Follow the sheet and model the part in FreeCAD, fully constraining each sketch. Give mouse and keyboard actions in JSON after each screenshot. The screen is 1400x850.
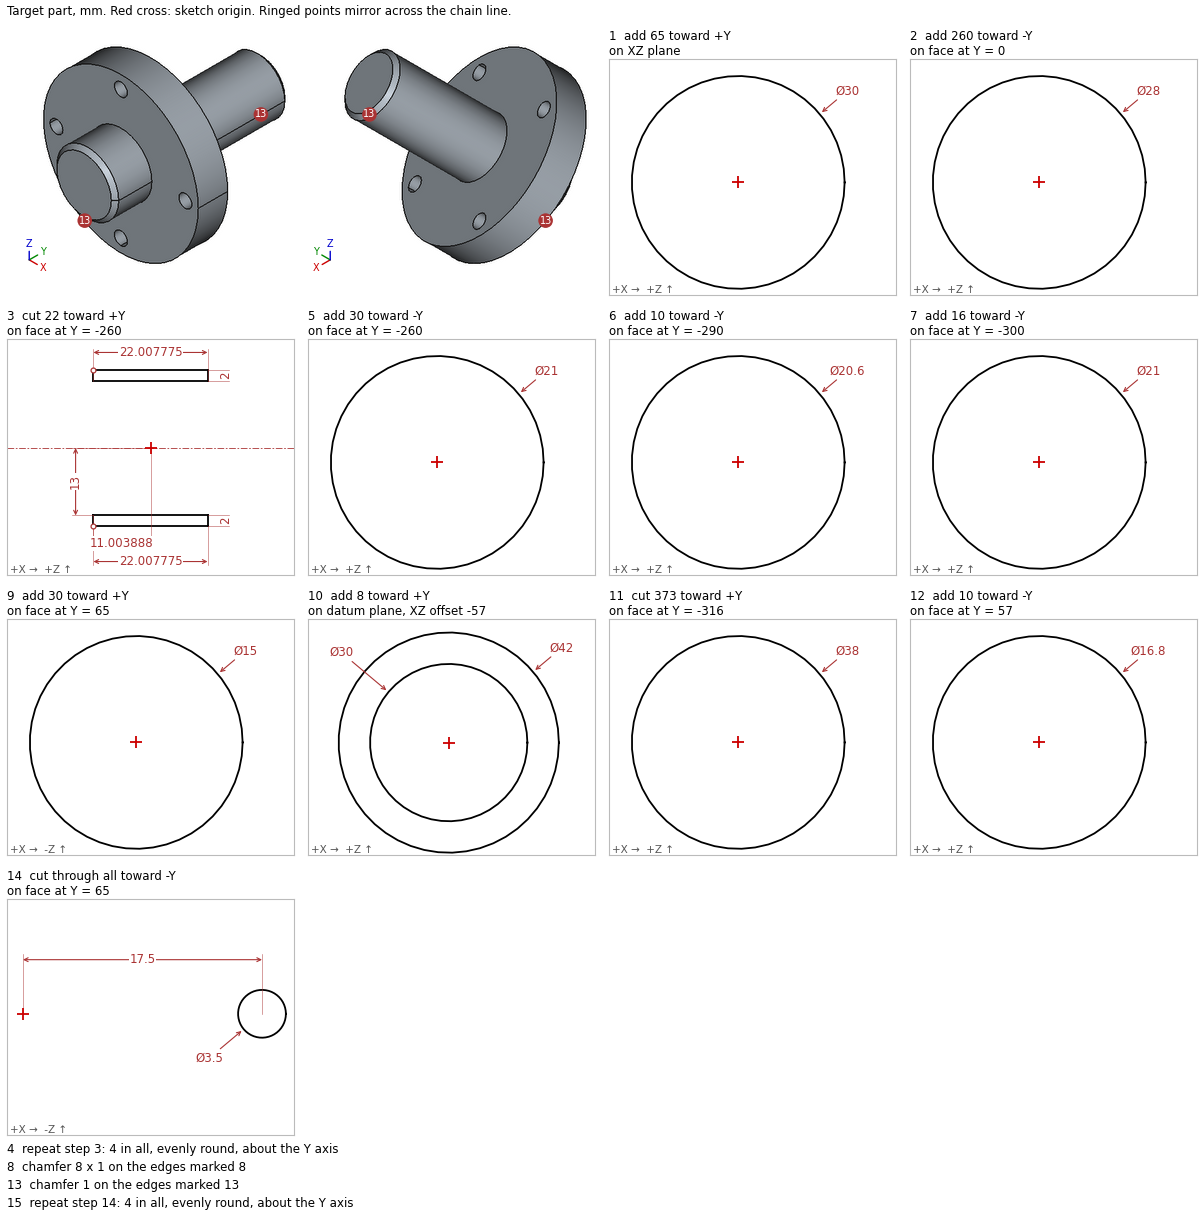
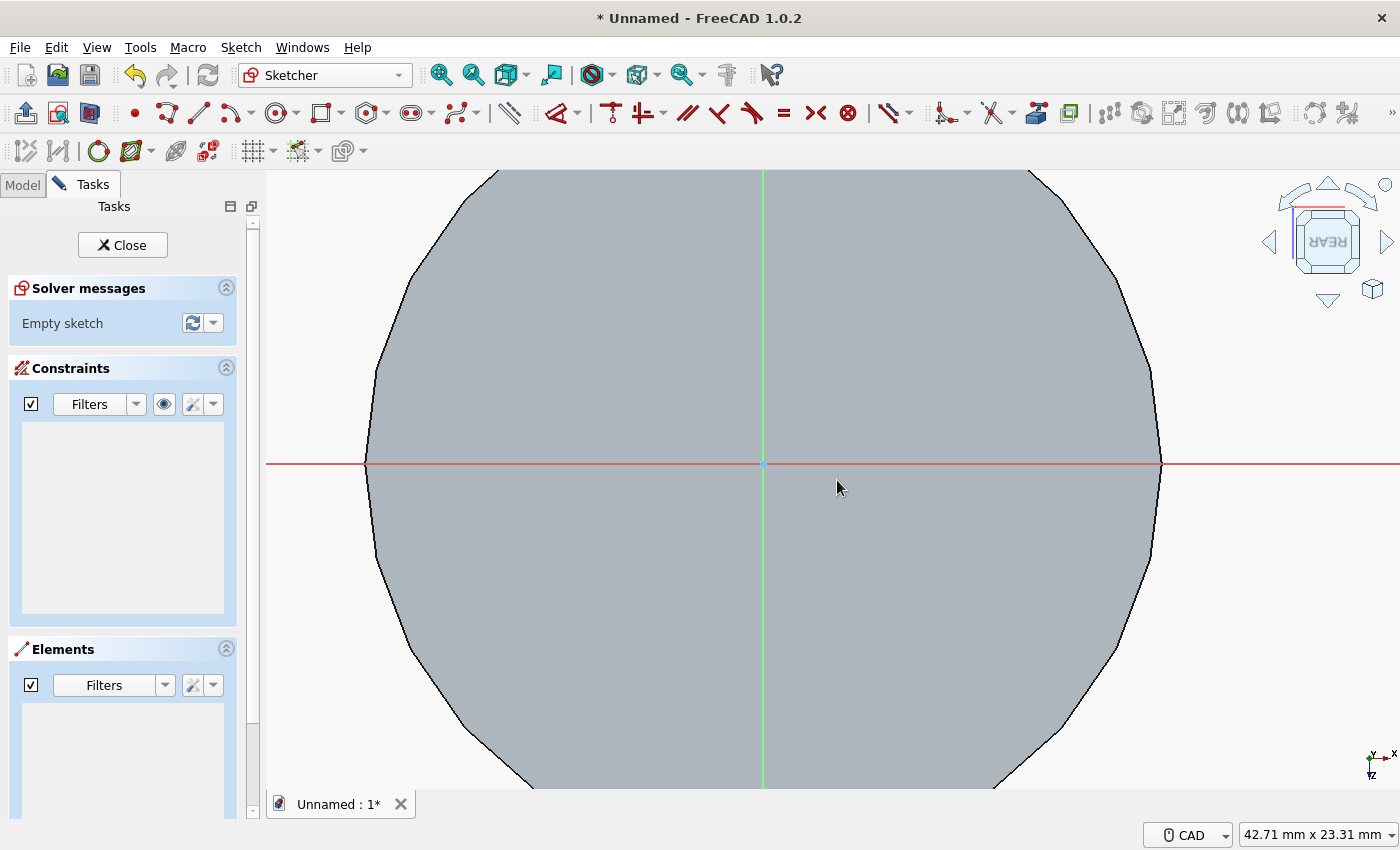
{"action": "key", "text": "g c"}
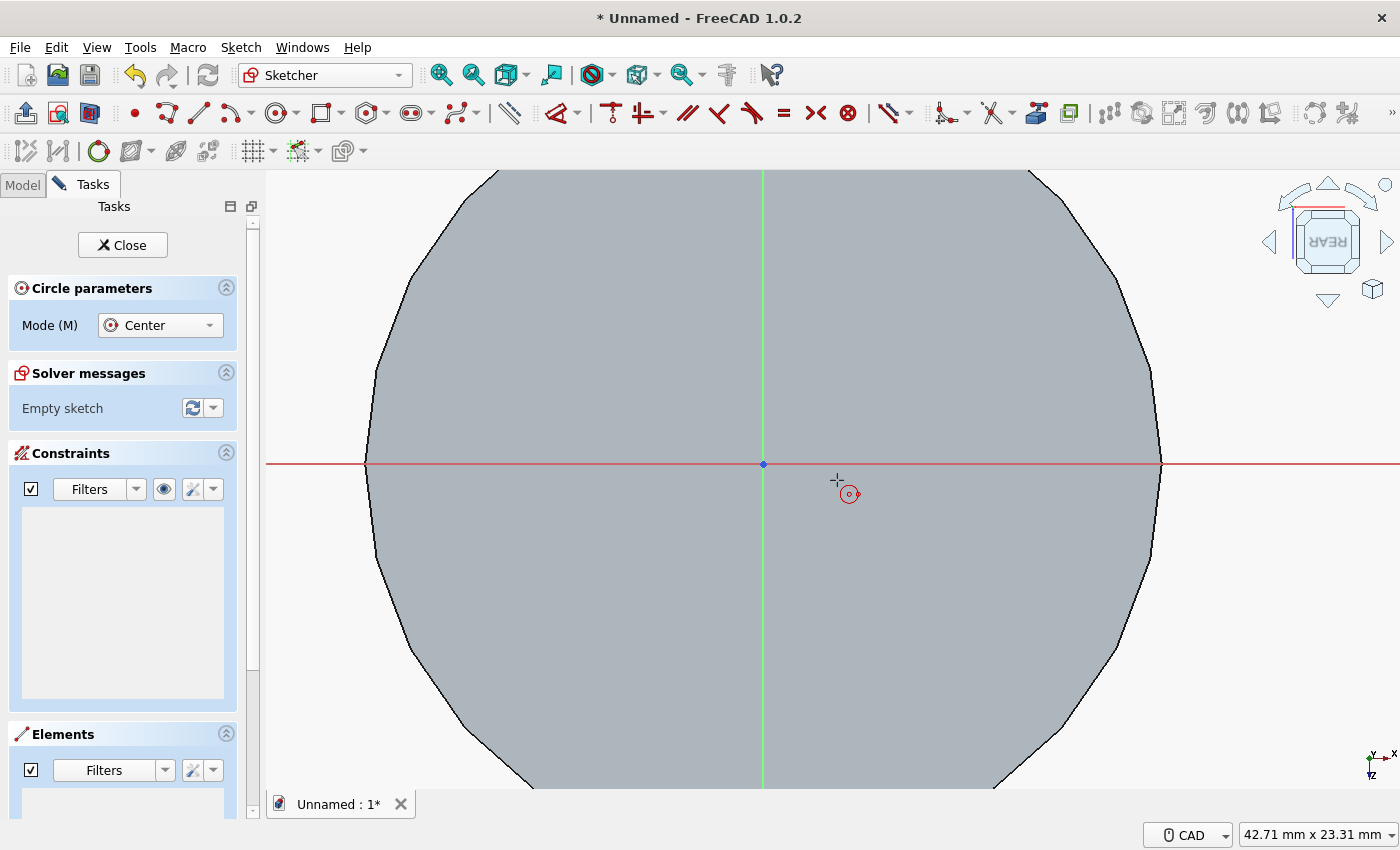
{"action": "left_click", "coordinate": [763, 464]}
{"action": "mouse_move", "coordinate": [904, 323]}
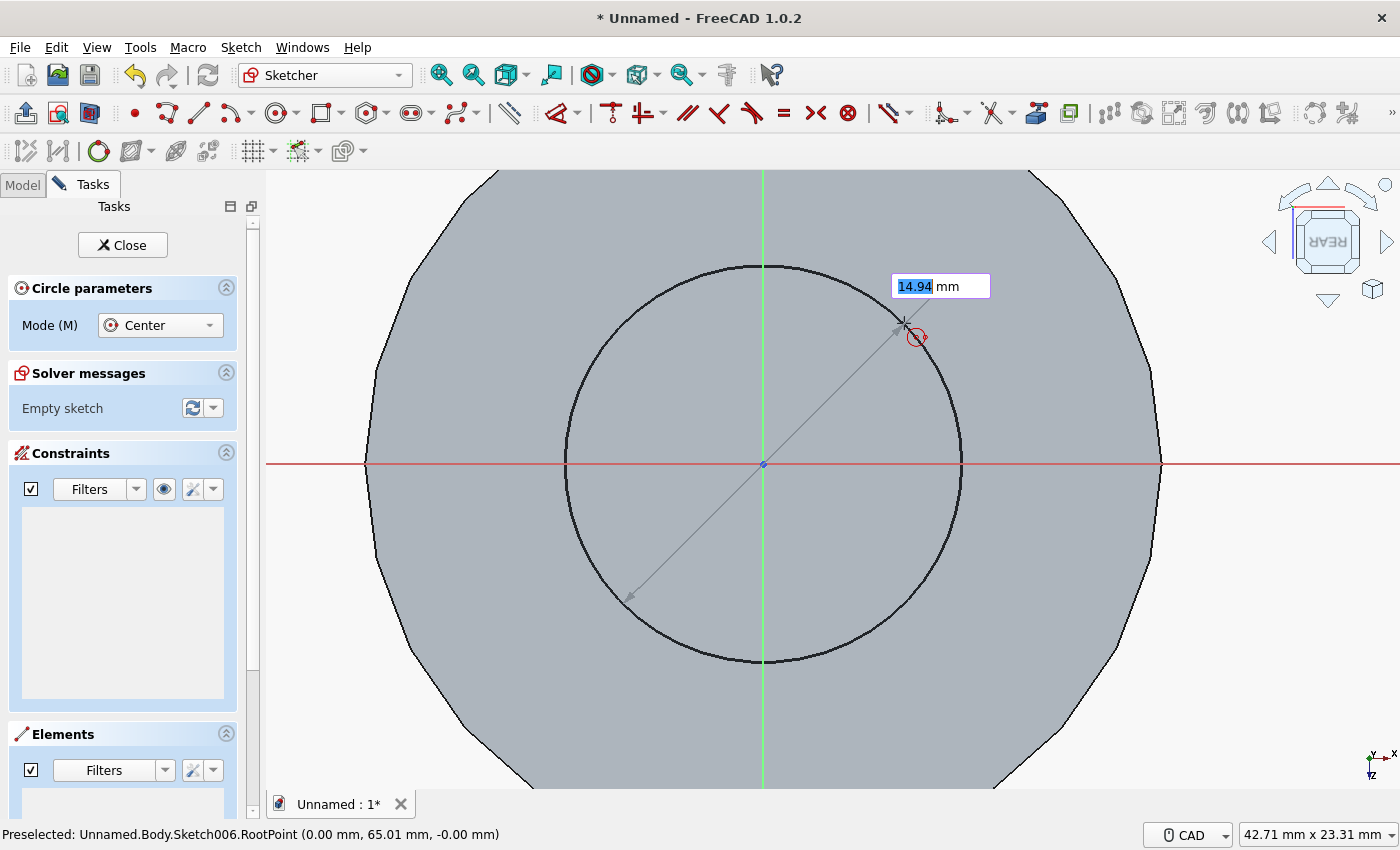
{"action": "type", "text": "15"}
{"action": "key", "text": "Return"}
{"action": "key", "text": "Escape"}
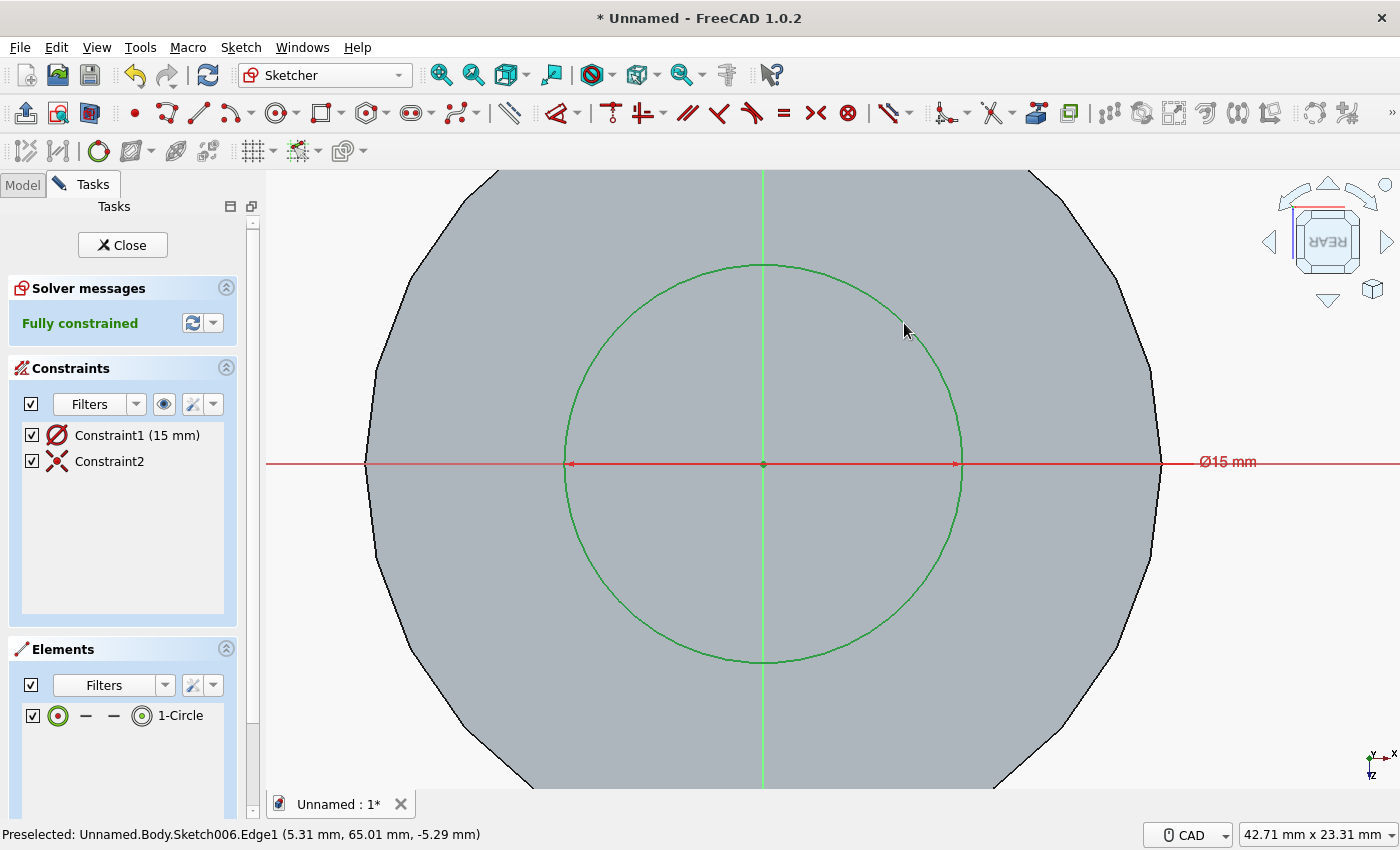
{"action": "left_click", "coordinate": [123, 245]}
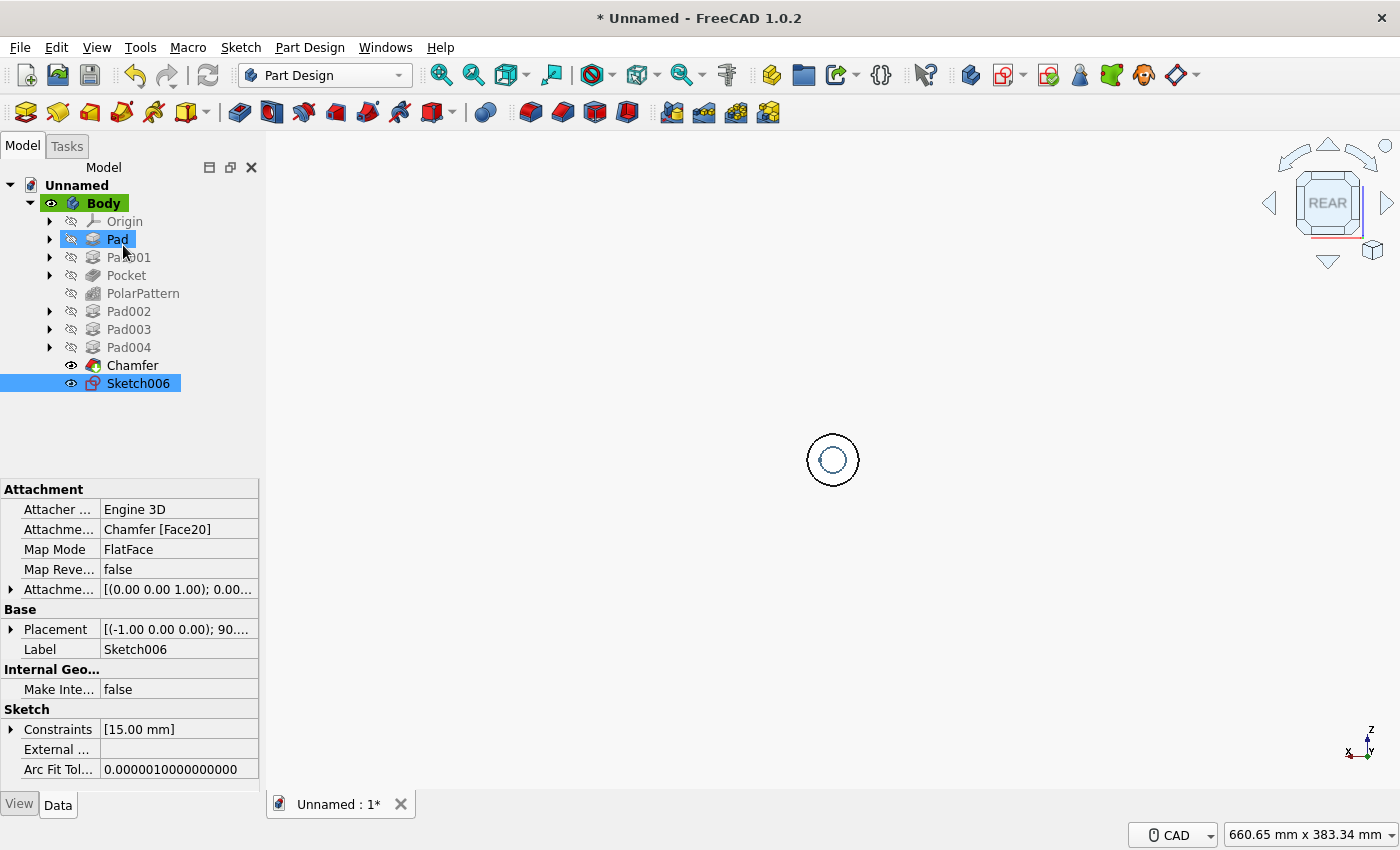
{"action": "left_click", "coordinate": [26, 112]}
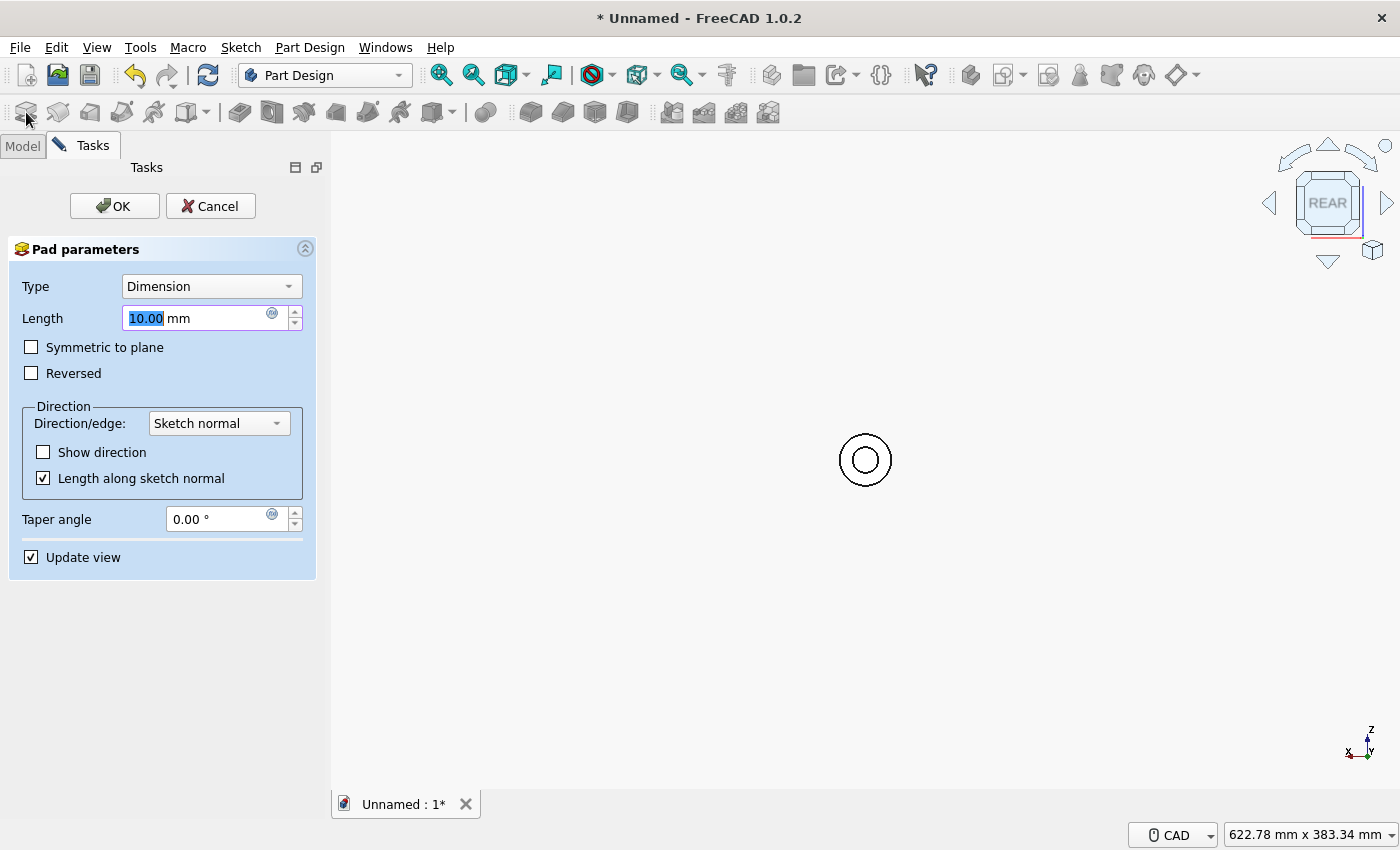
{"action": "type", "text": "30"}
{"action": "key", "text": "Tab"}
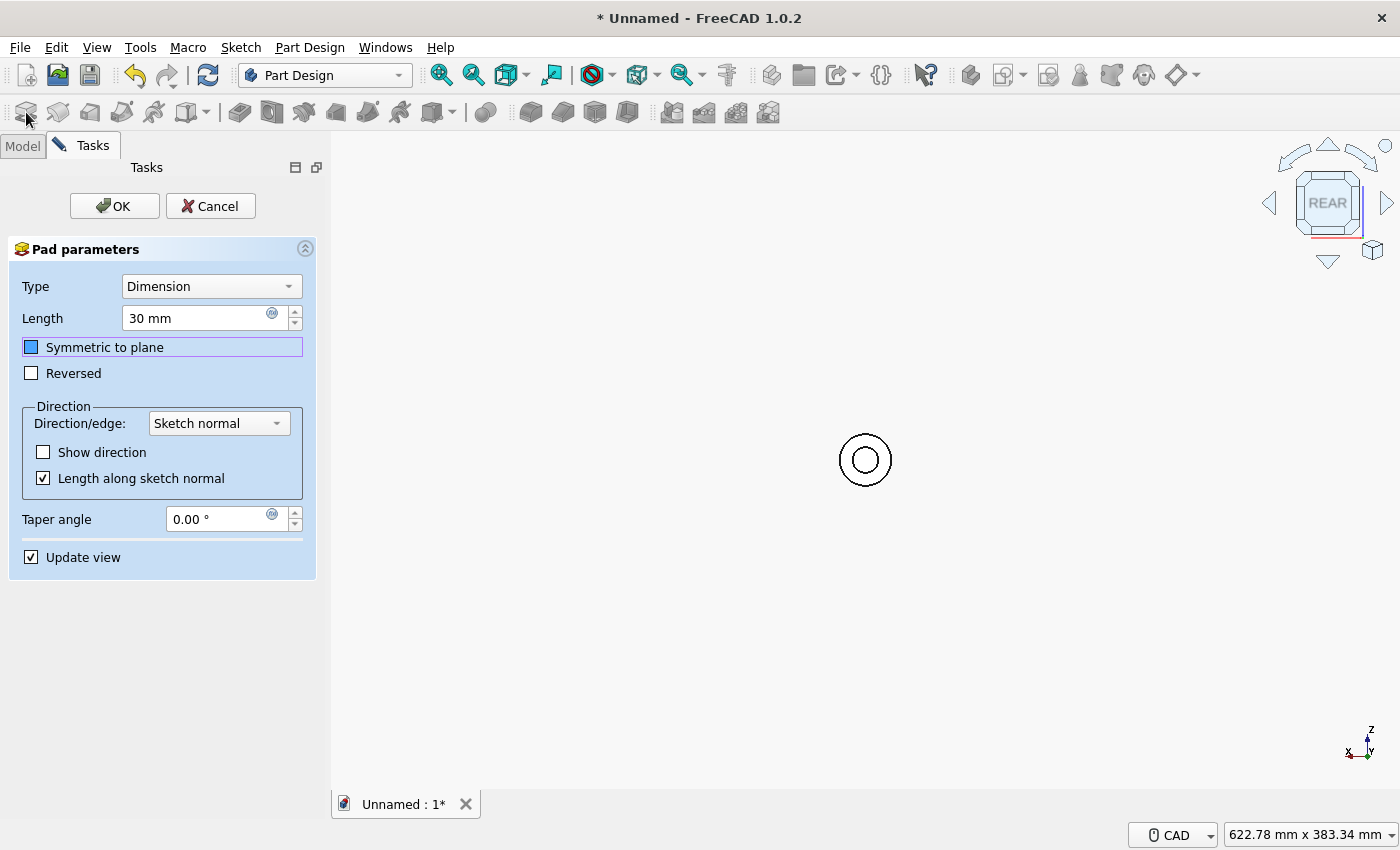
{"action": "left_click", "coordinate": [115, 206]}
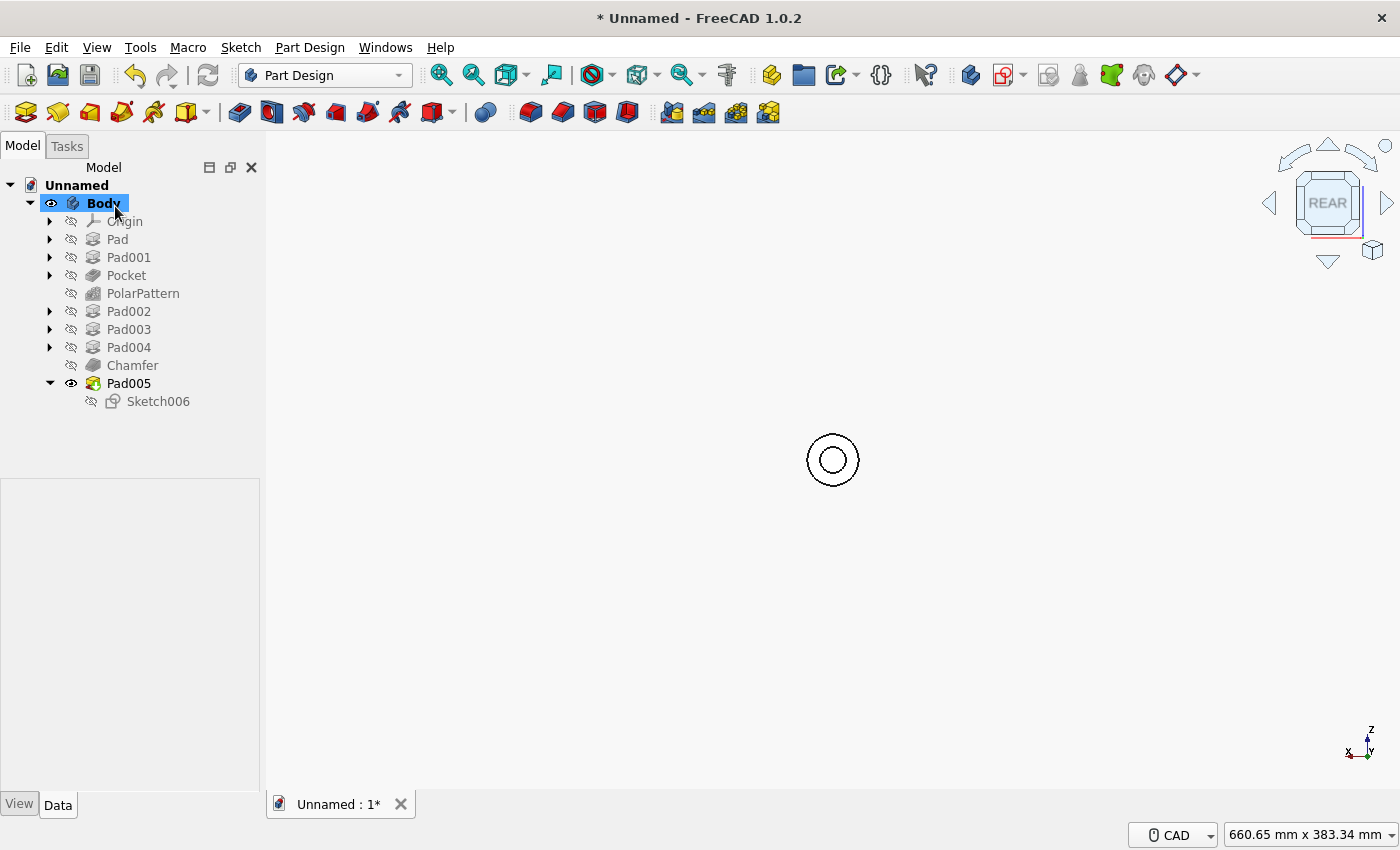
{"action": "left_click", "coordinate": [442, 76]}